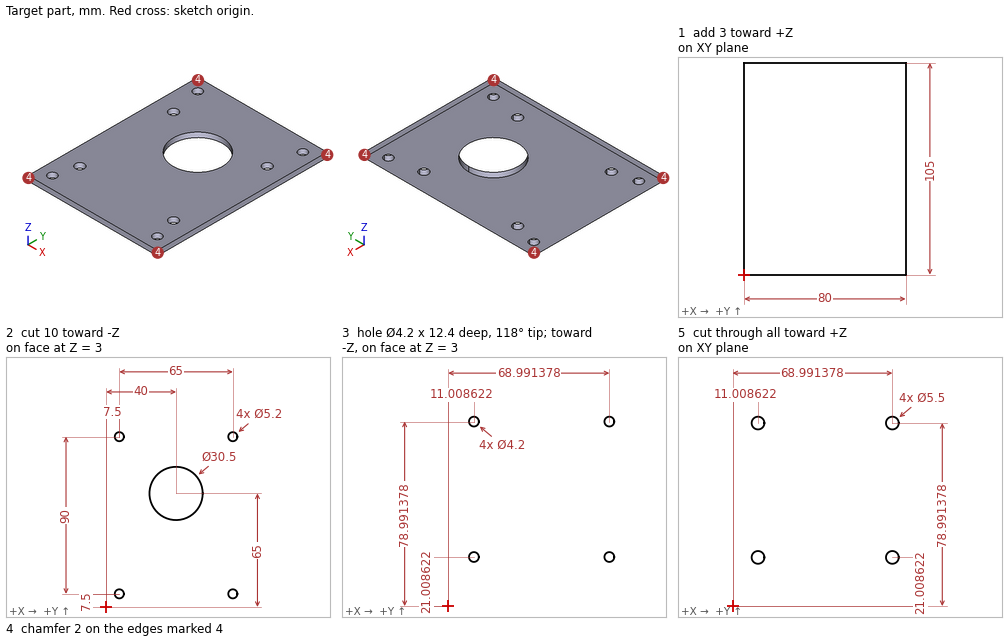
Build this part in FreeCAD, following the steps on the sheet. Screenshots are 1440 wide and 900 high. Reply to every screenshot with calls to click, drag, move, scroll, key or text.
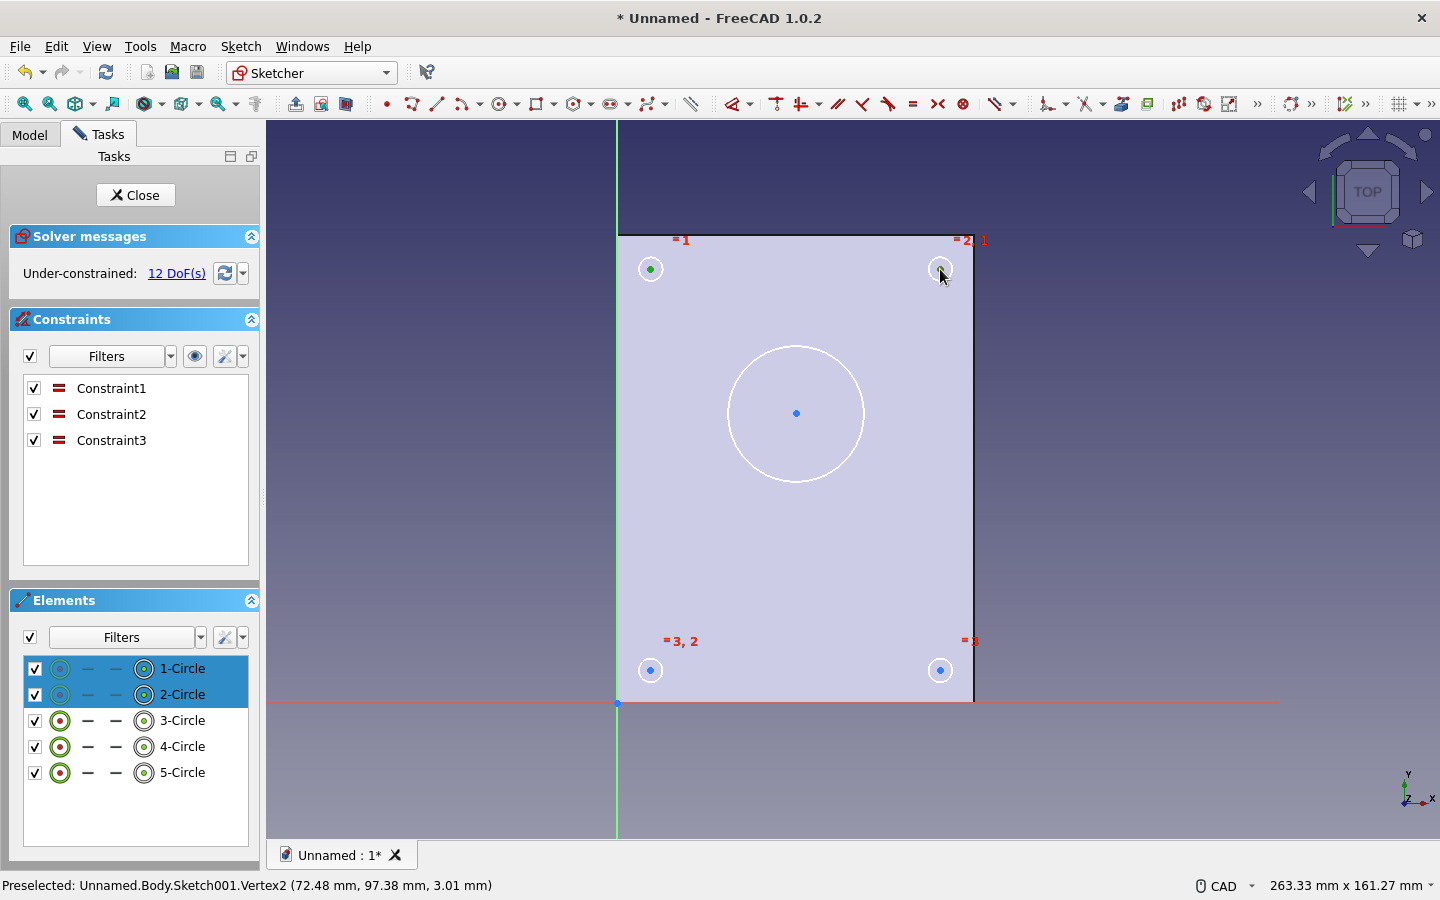
key(h)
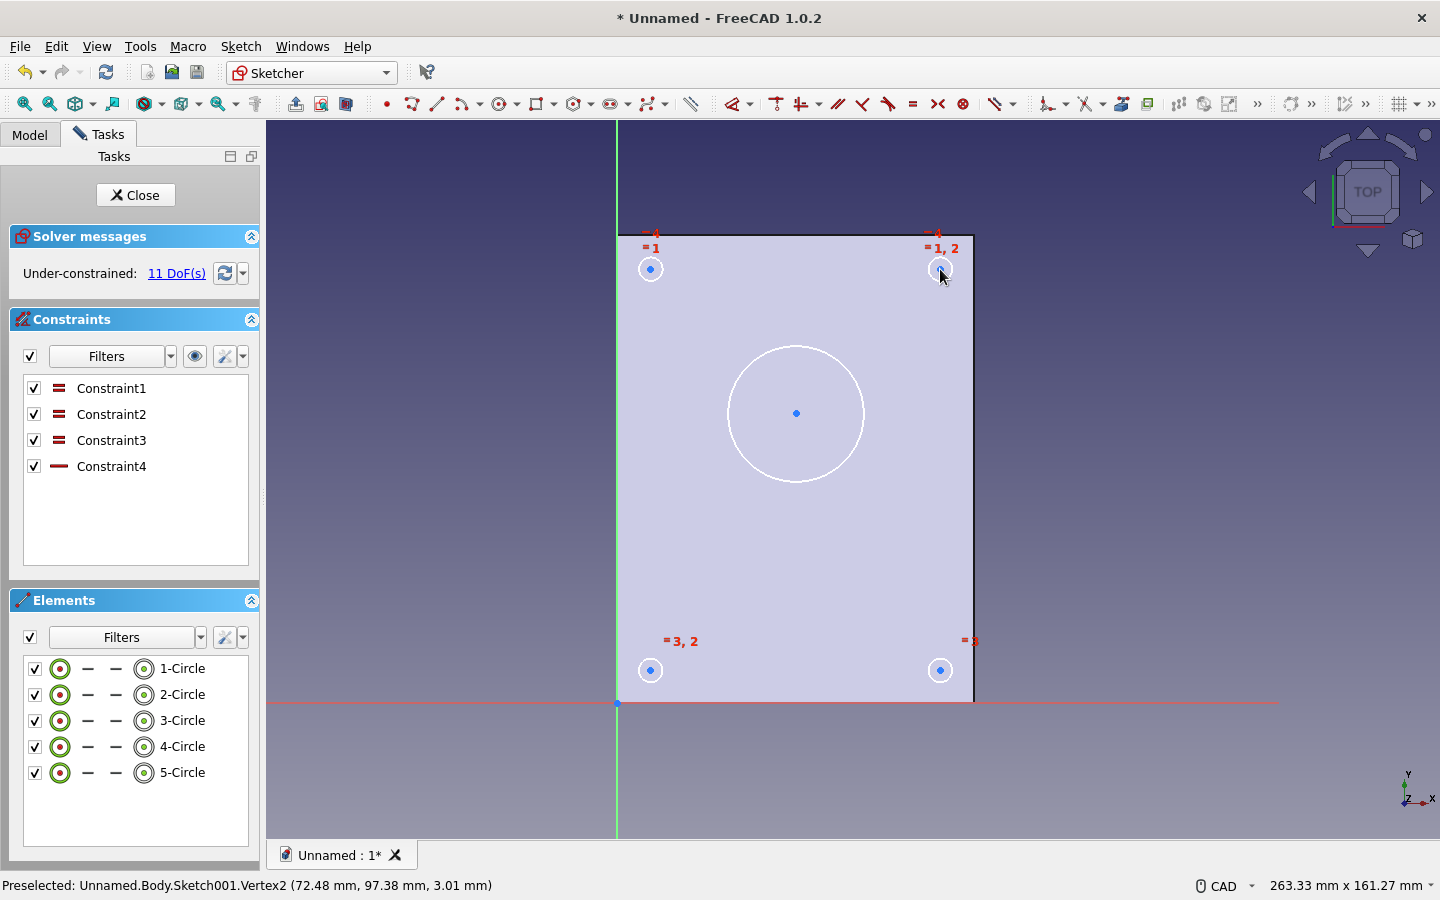
click(651, 269)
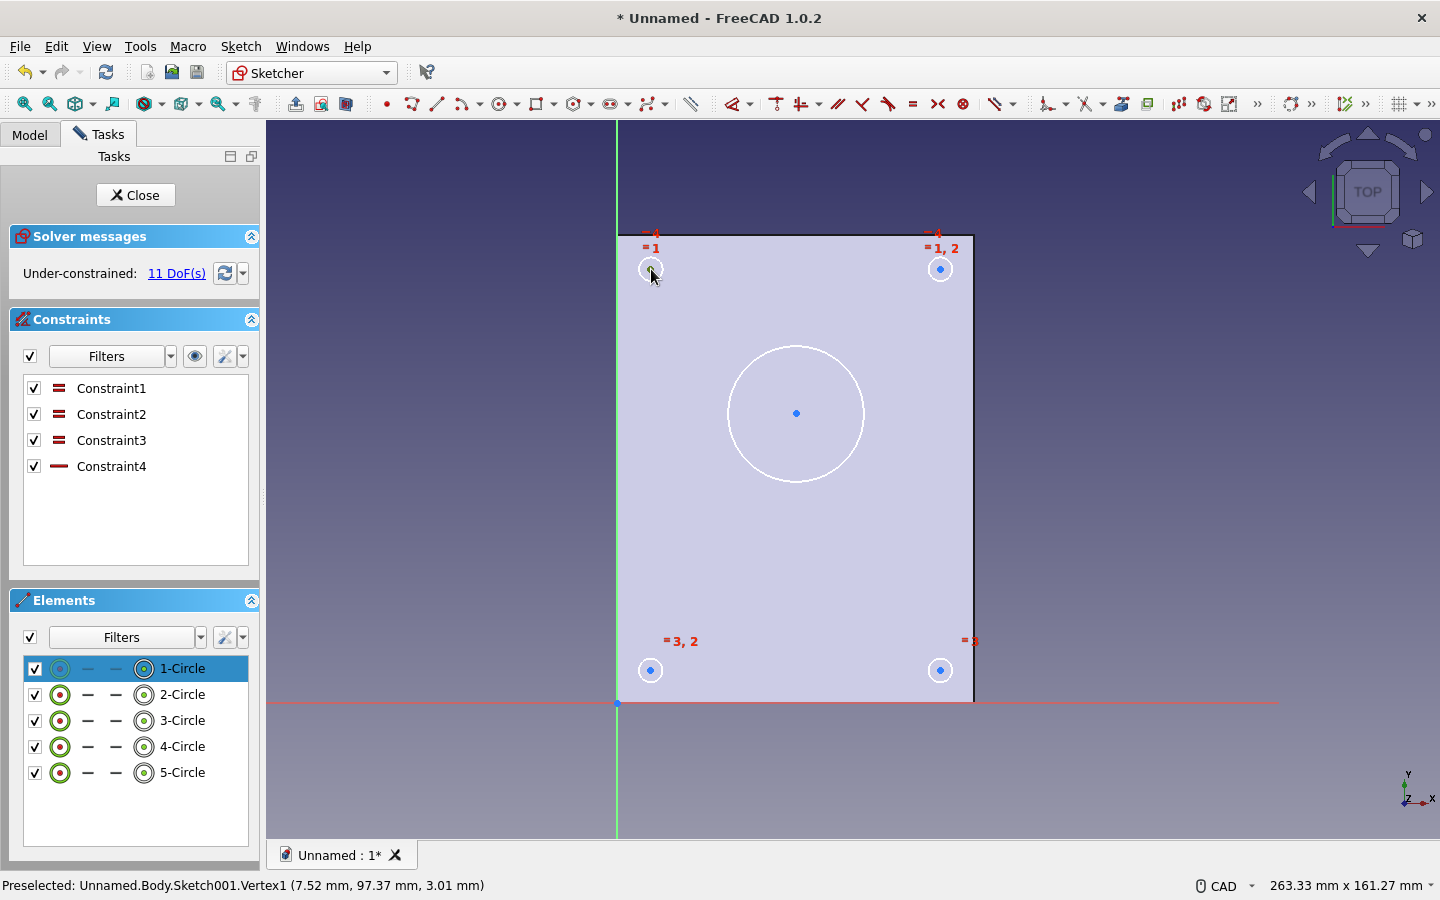
click(651, 670)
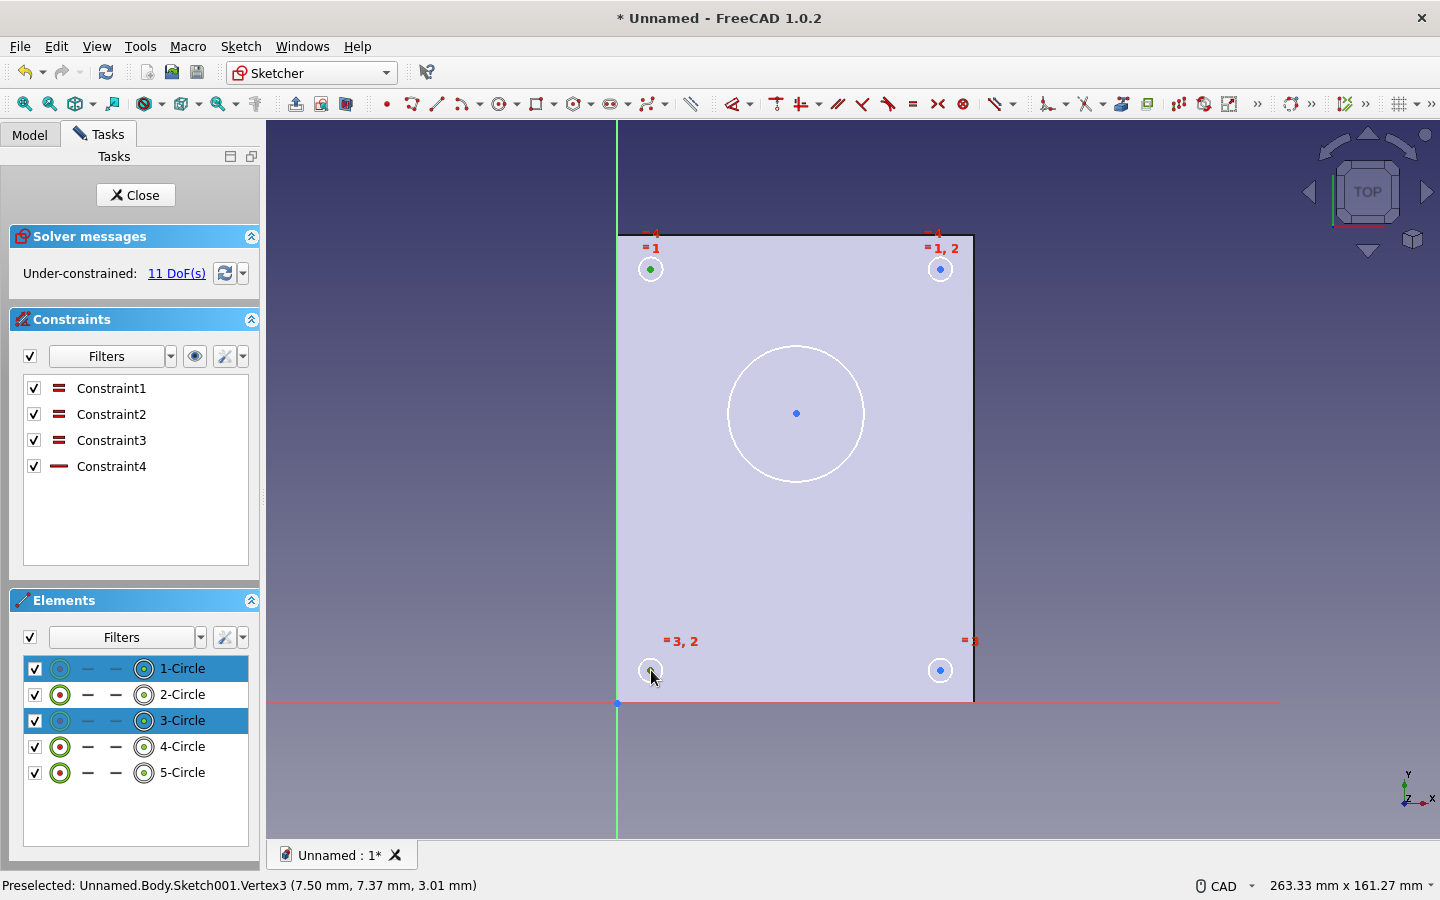
click(818, 104)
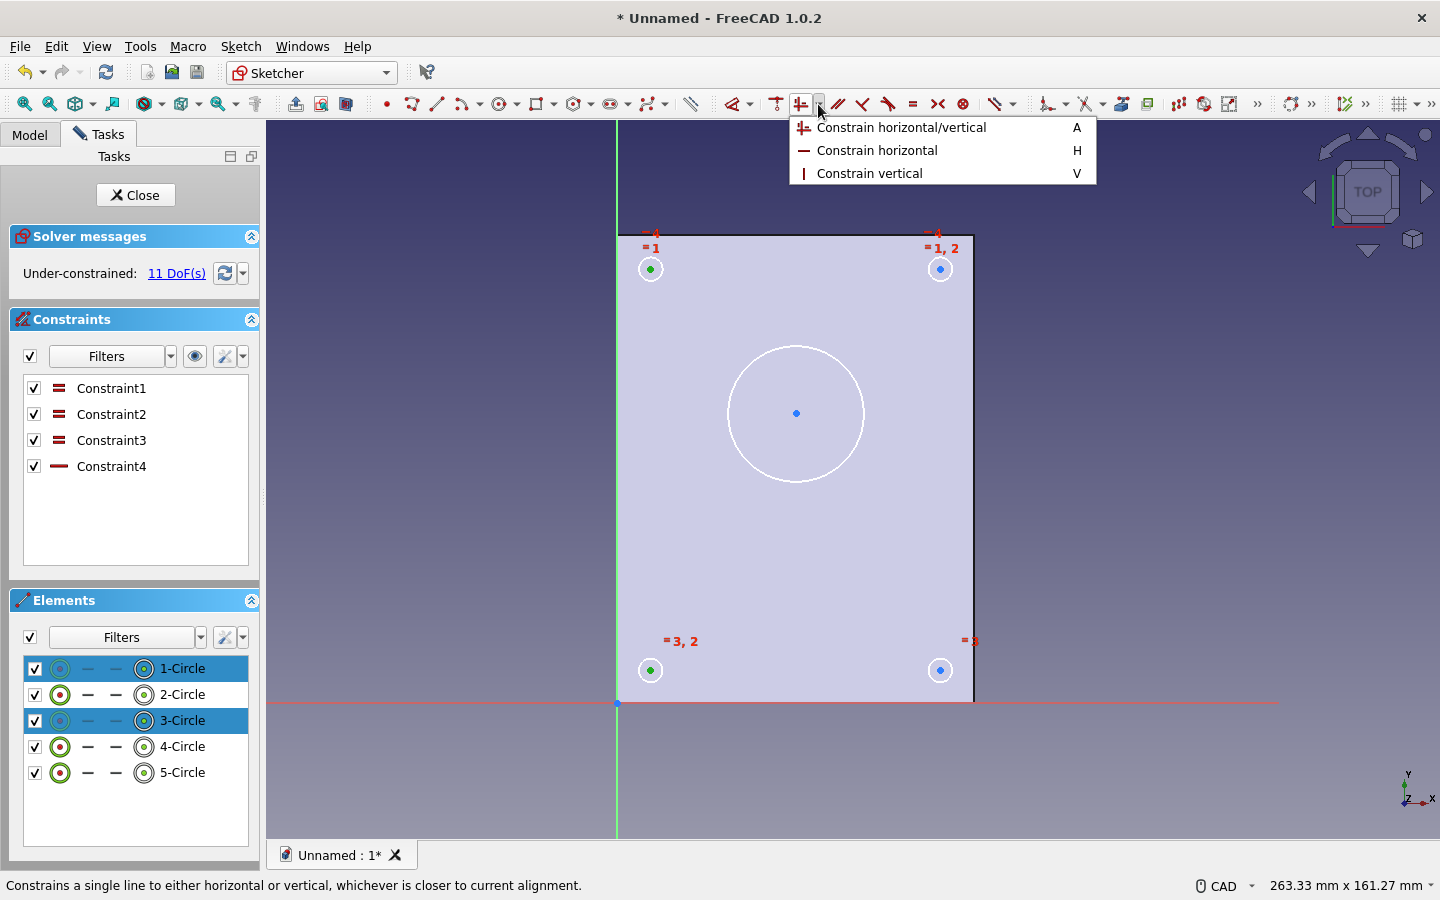
click(943, 174)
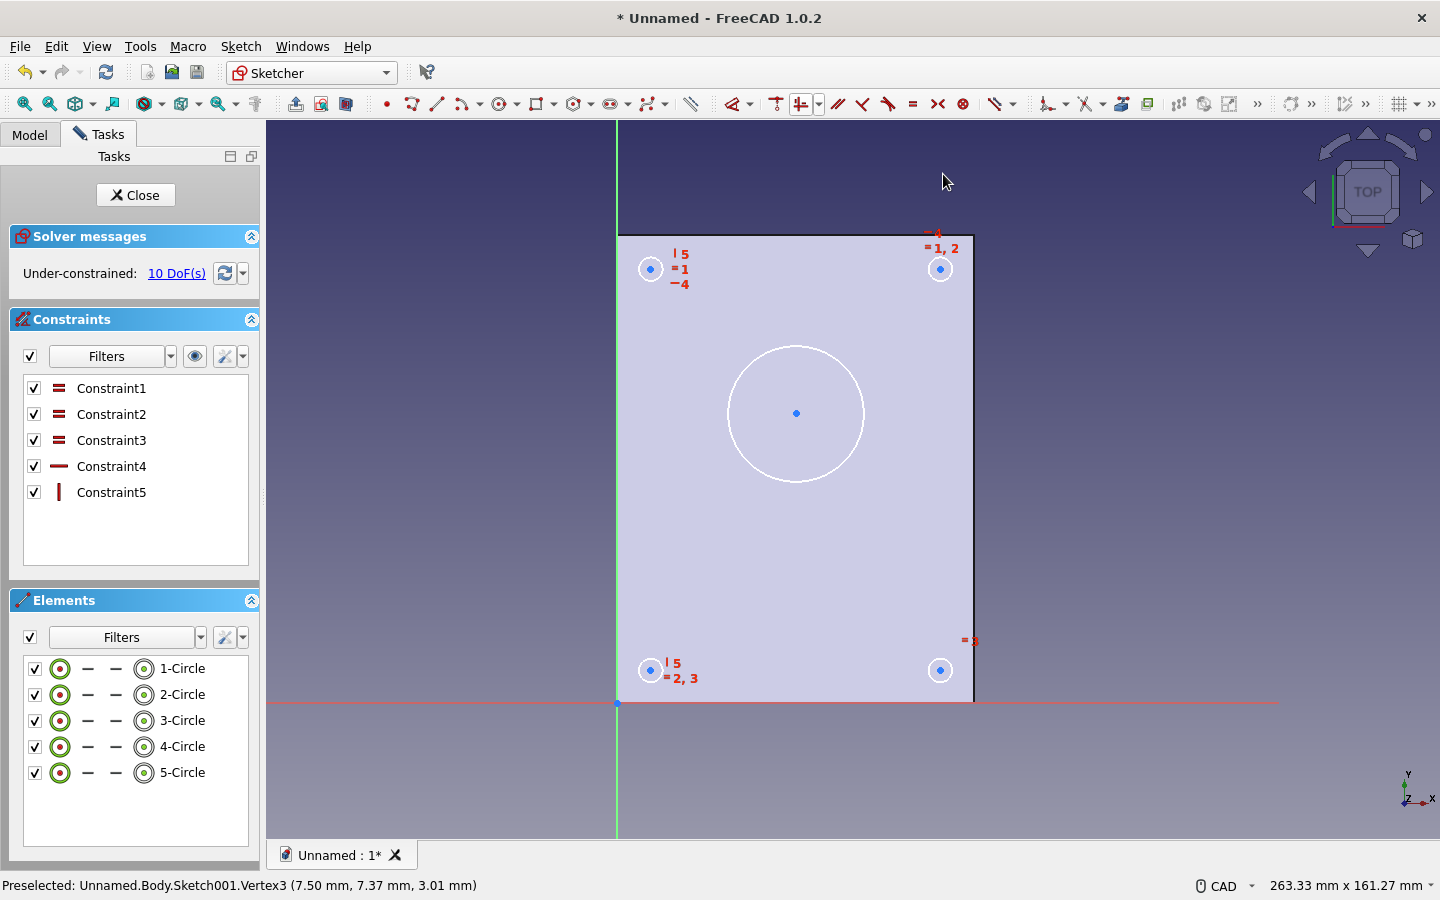
click(940, 269)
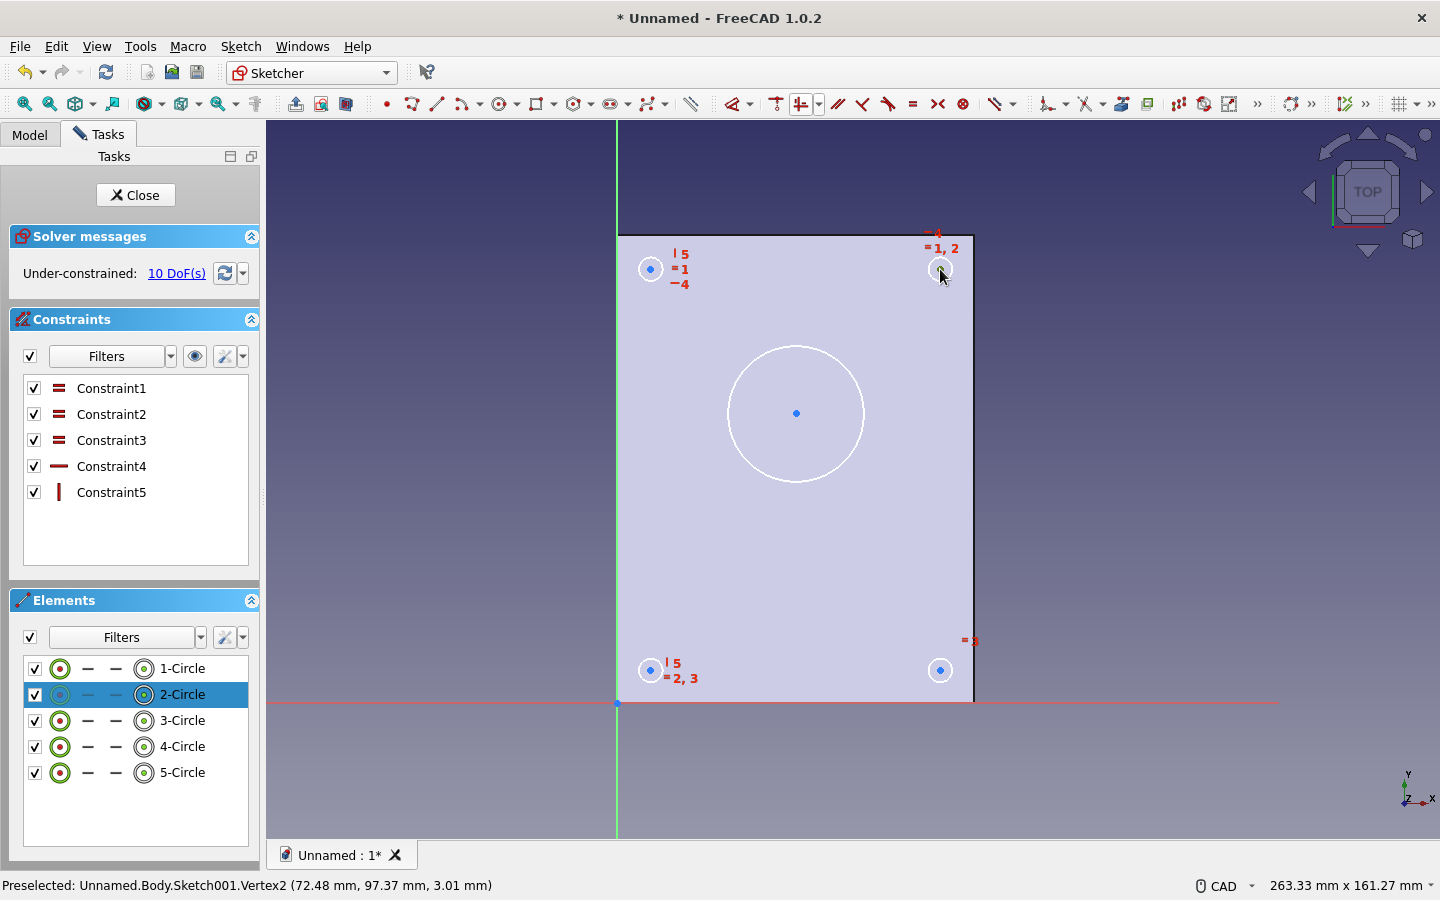
click(940, 670)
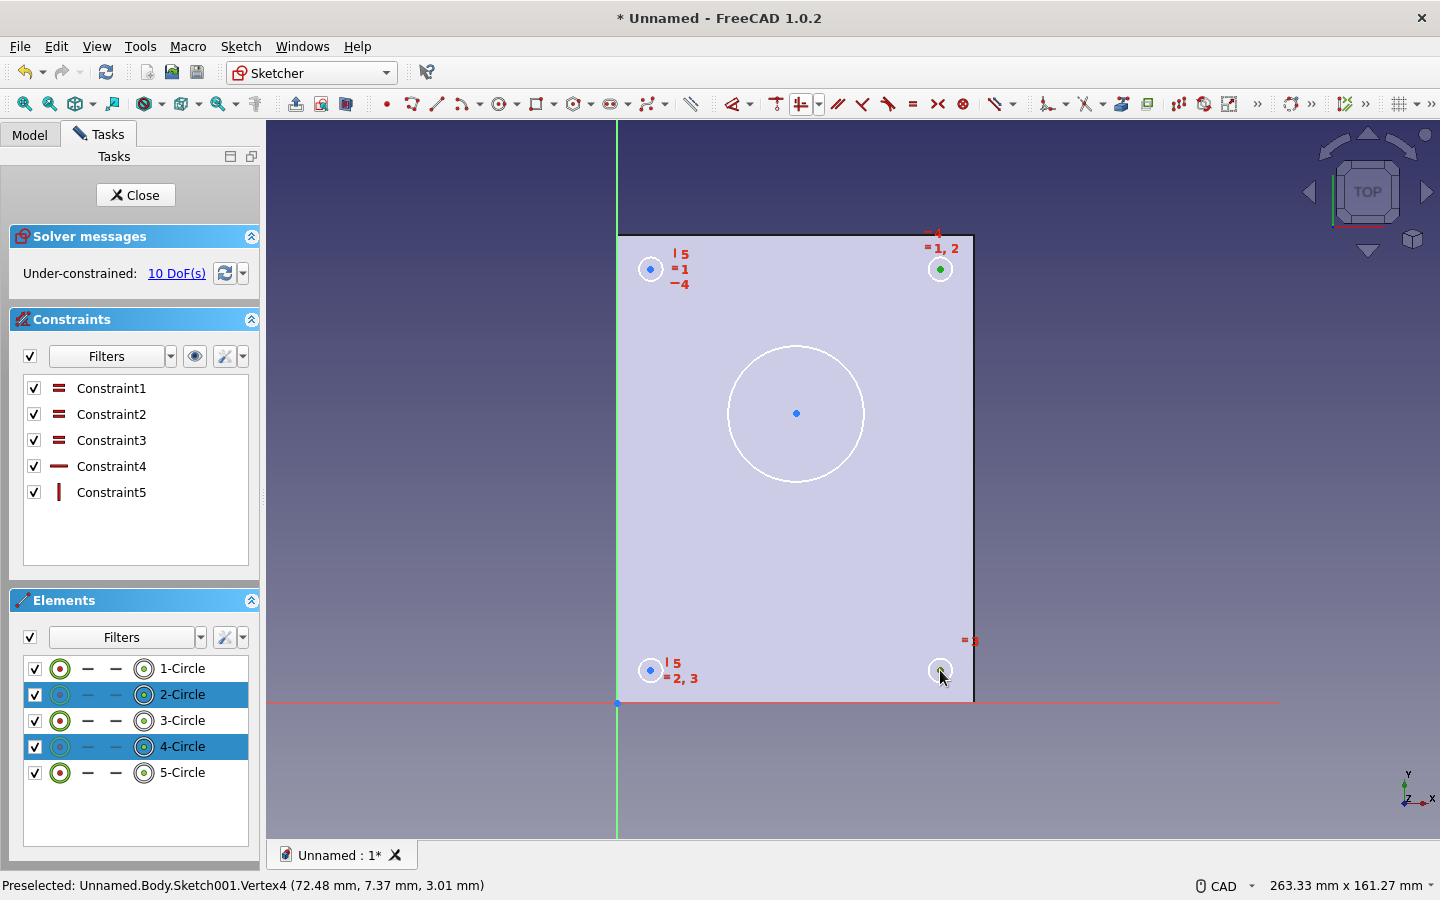
click(818, 104)